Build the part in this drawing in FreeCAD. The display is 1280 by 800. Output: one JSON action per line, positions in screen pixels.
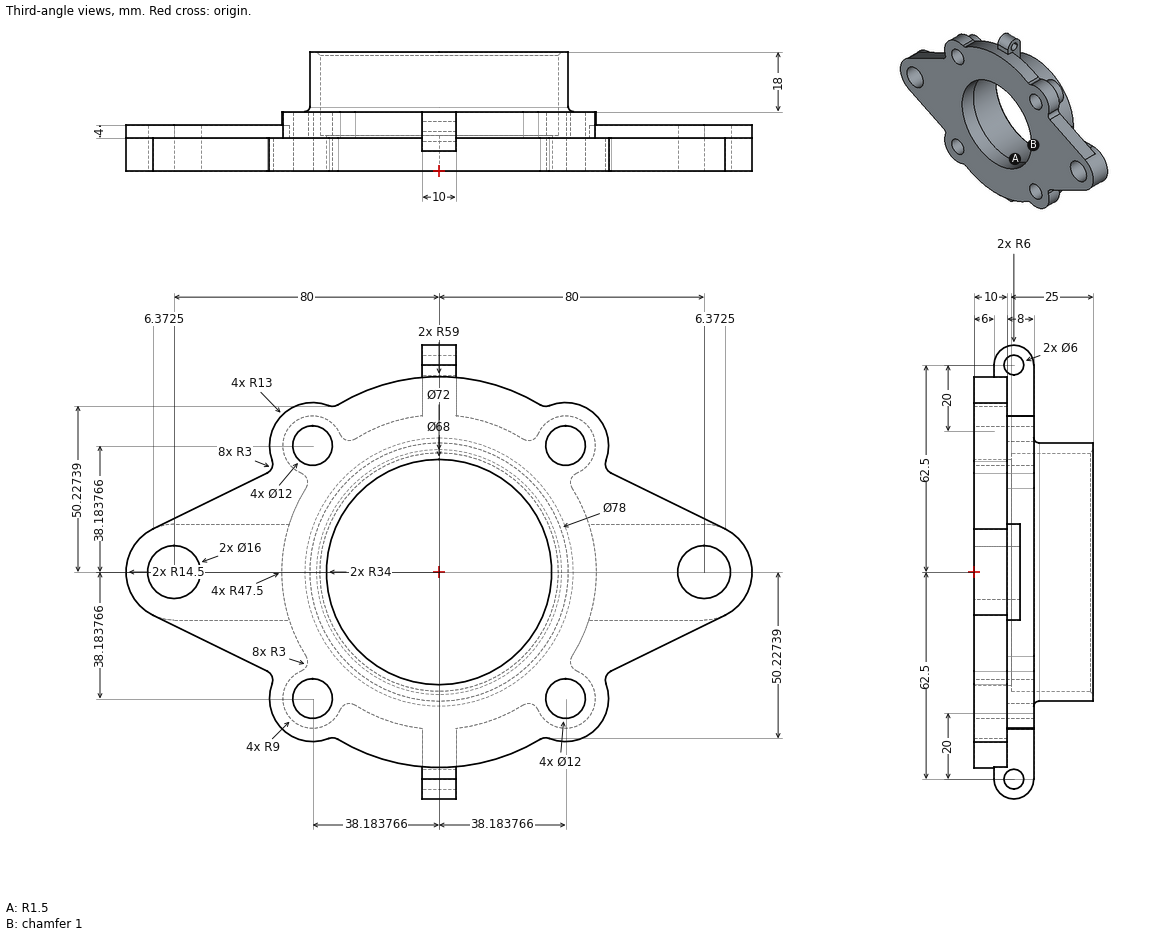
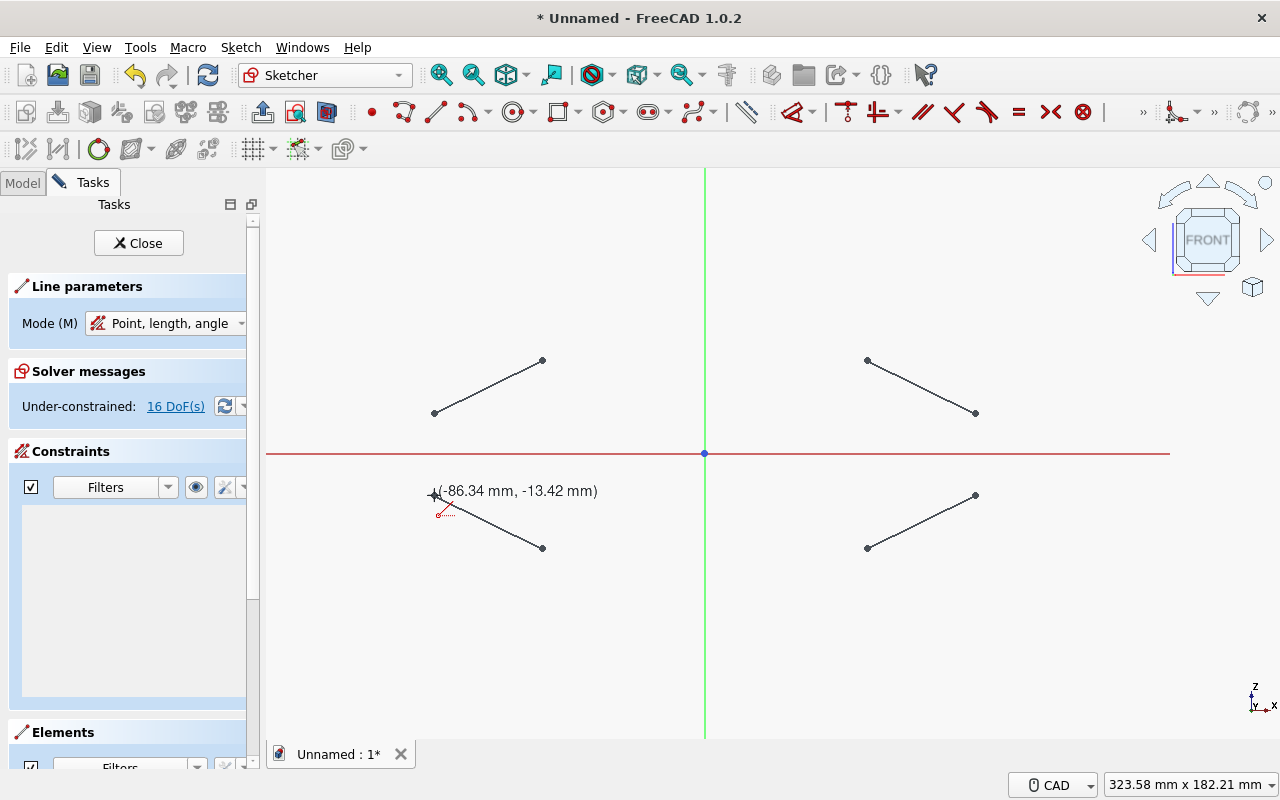
{"action": "left_click", "coordinate": [490, 112]}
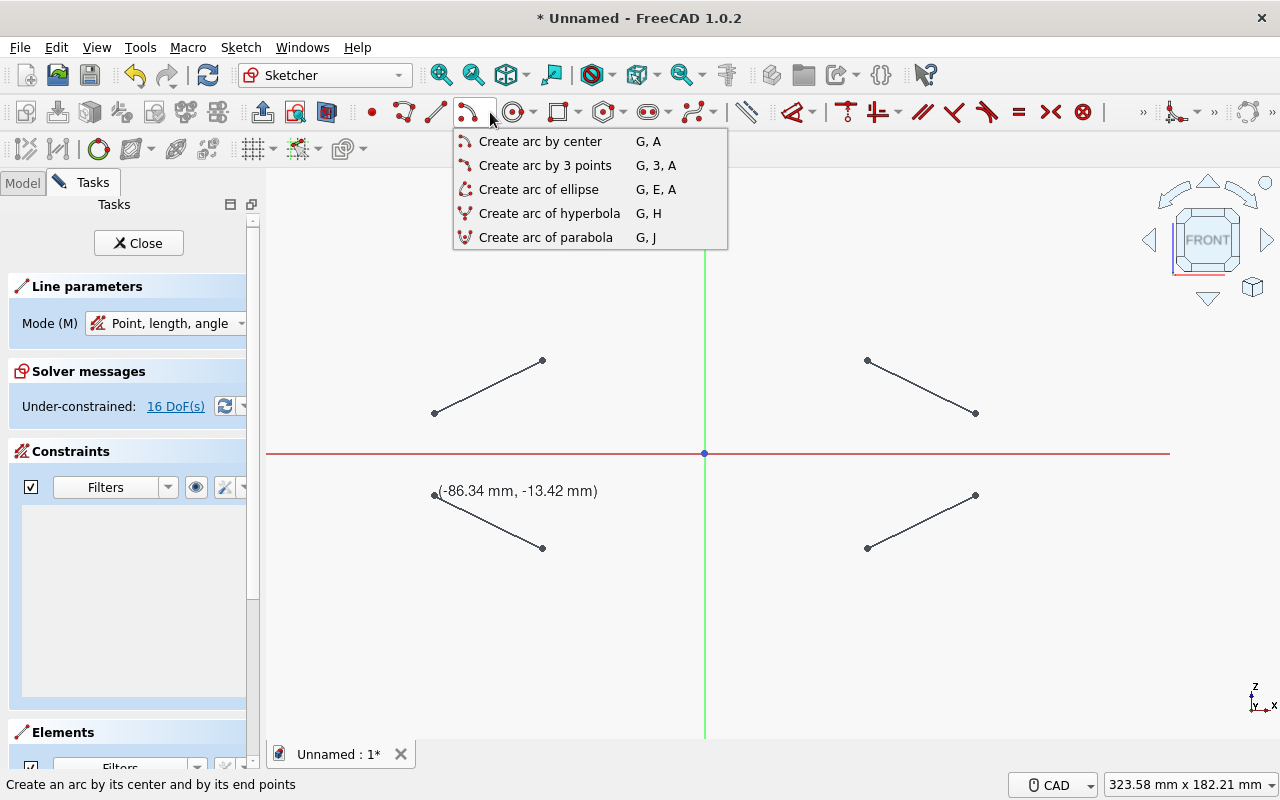
{"action": "left_click", "coordinate": [590, 165]}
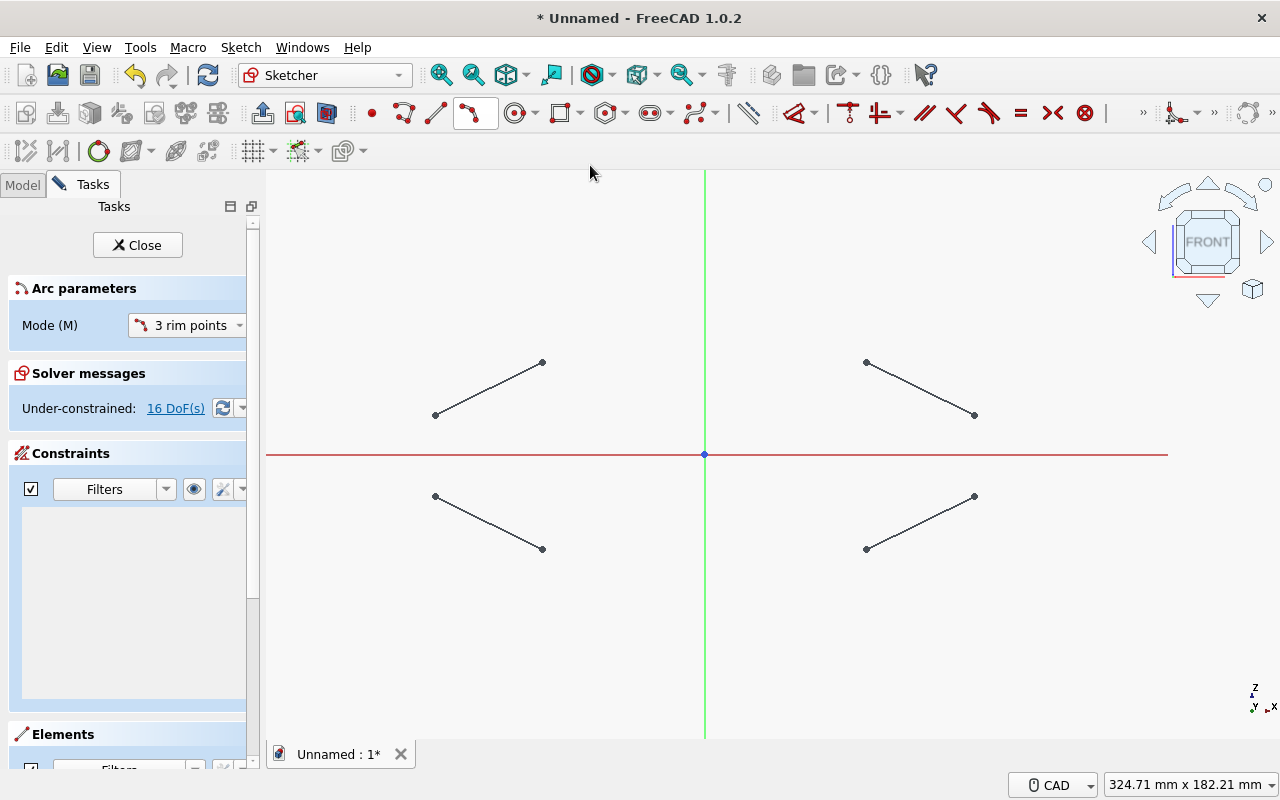
{"action": "left_click", "coordinate": [543, 362]}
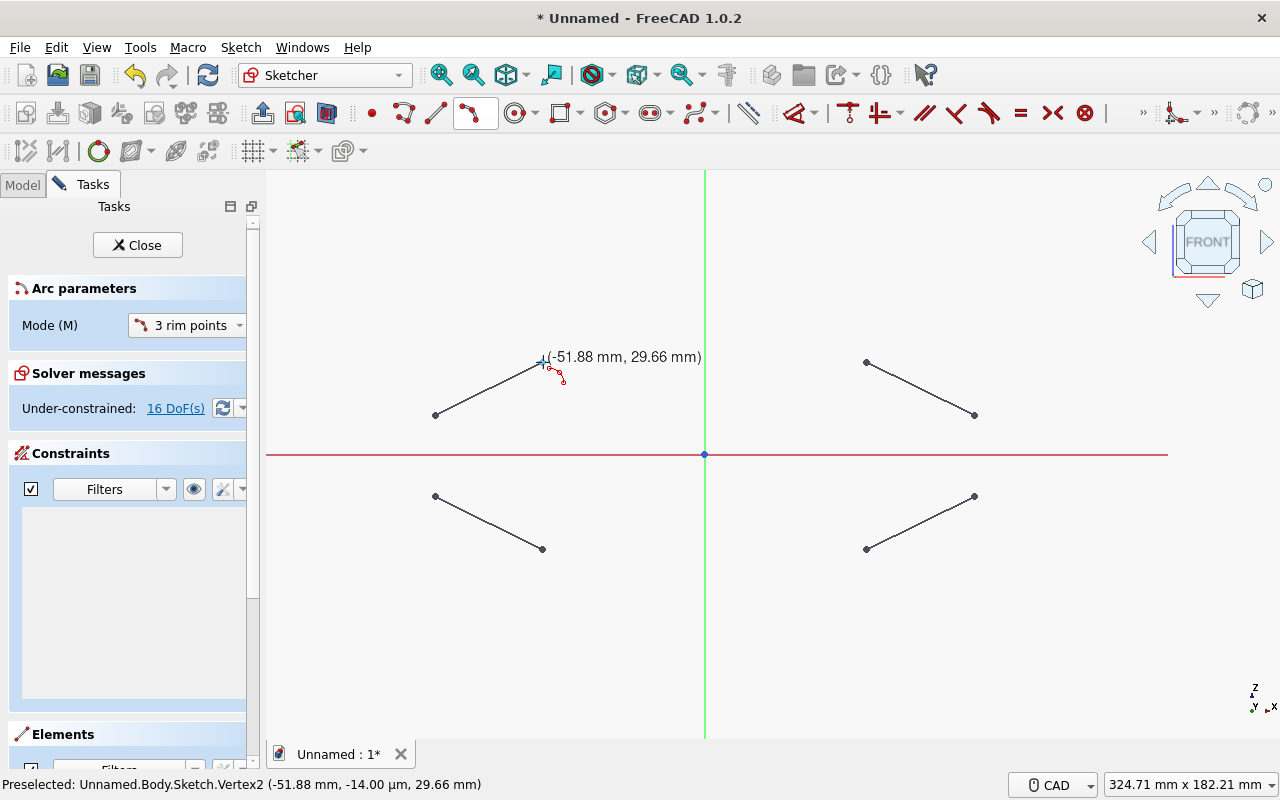
{"action": "scroll", "coordinate": [548, 350], "scroll_direction": "up", "scroll_amount": 2}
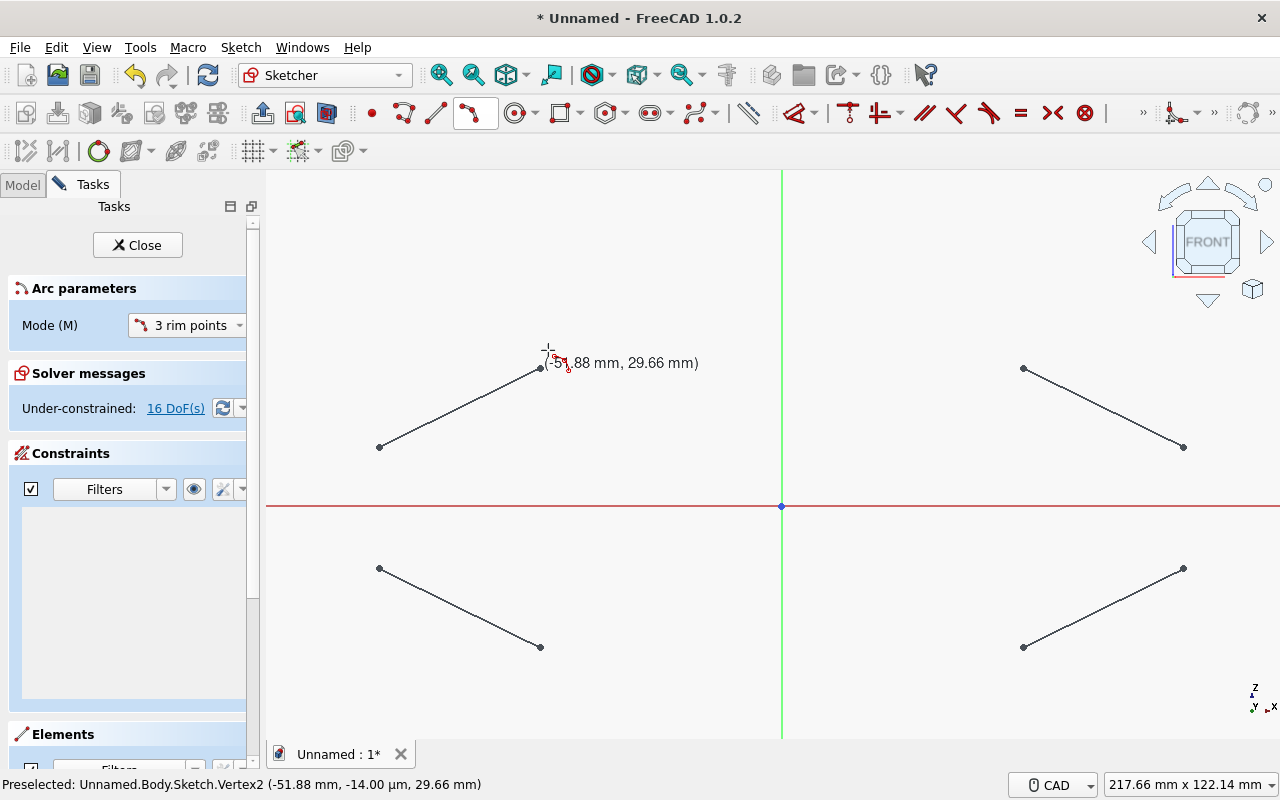
{"action": "left_click", "coordinate": [547, 350]}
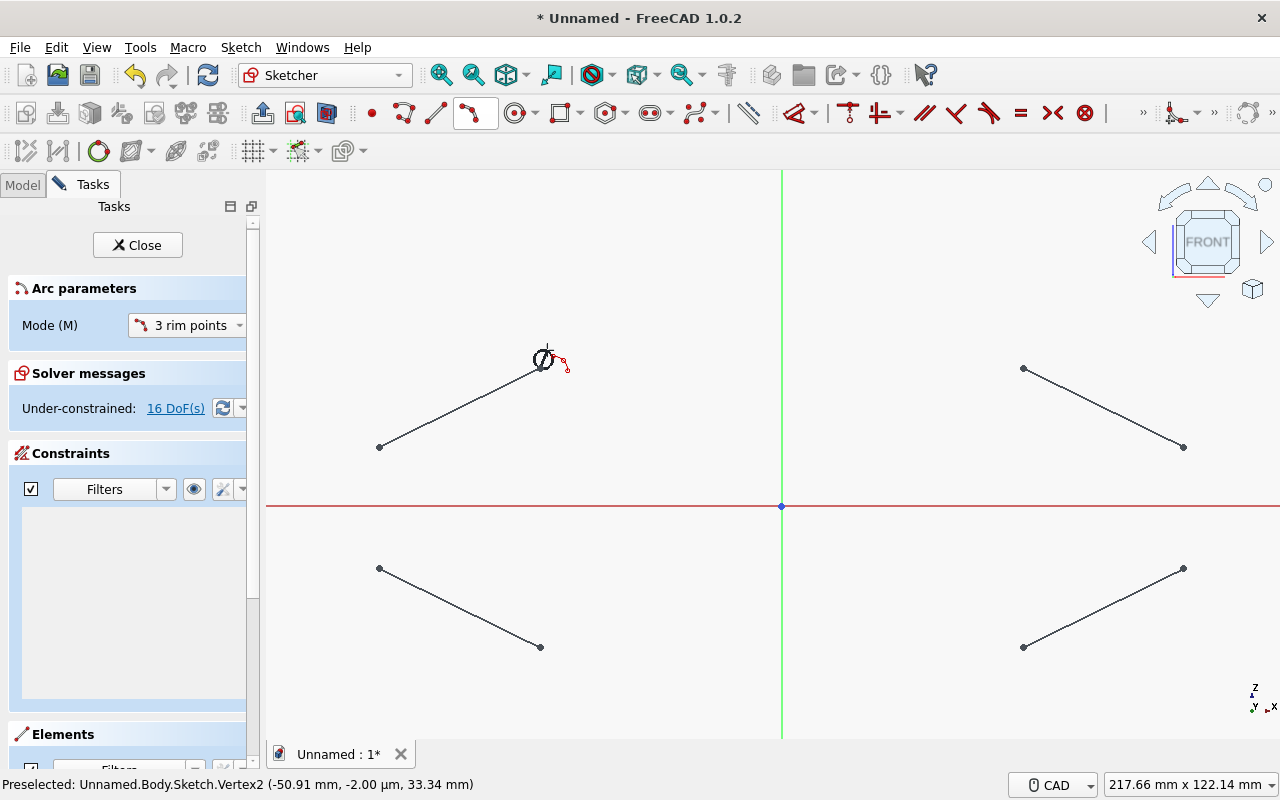
{"action": "scroll", "coordinate": [547, 360], "scroll_direction": "up", "scroll_amount": 8}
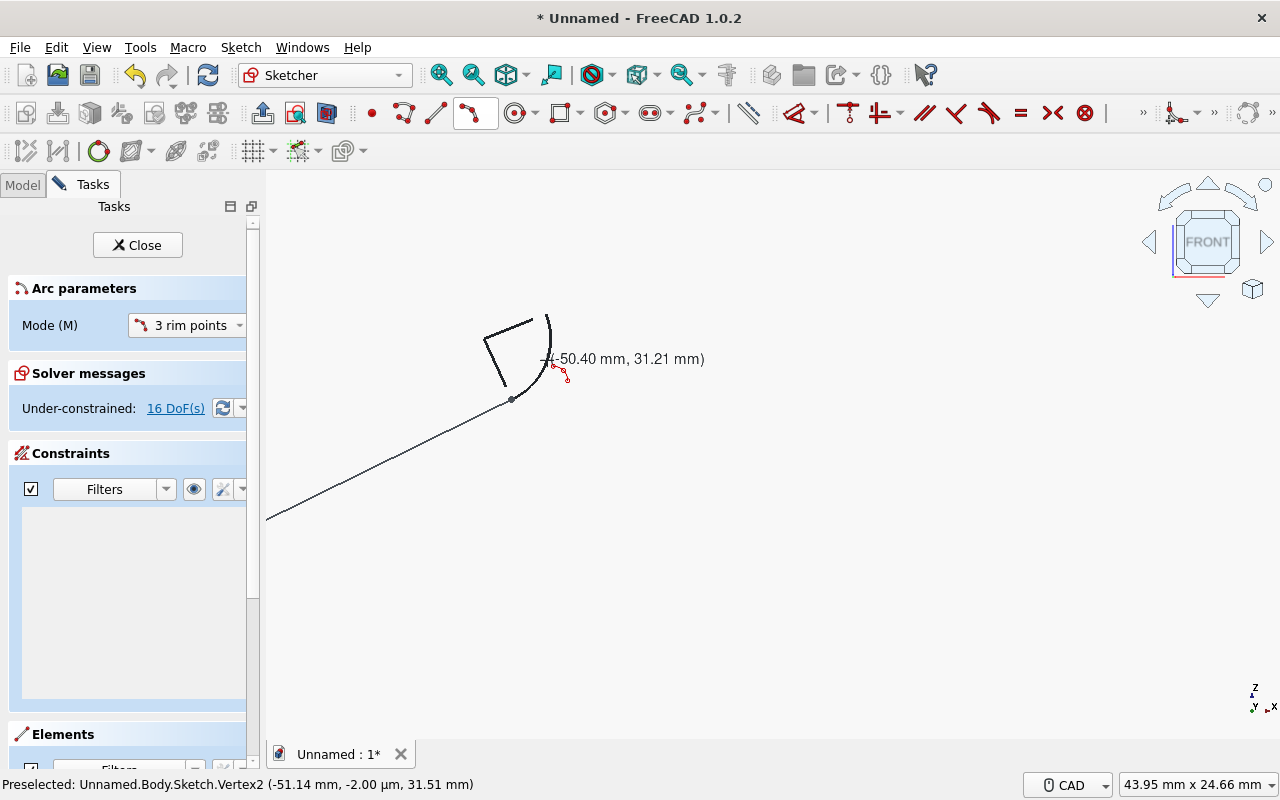
{"action": "left_click", "coordinate": [546, 357]}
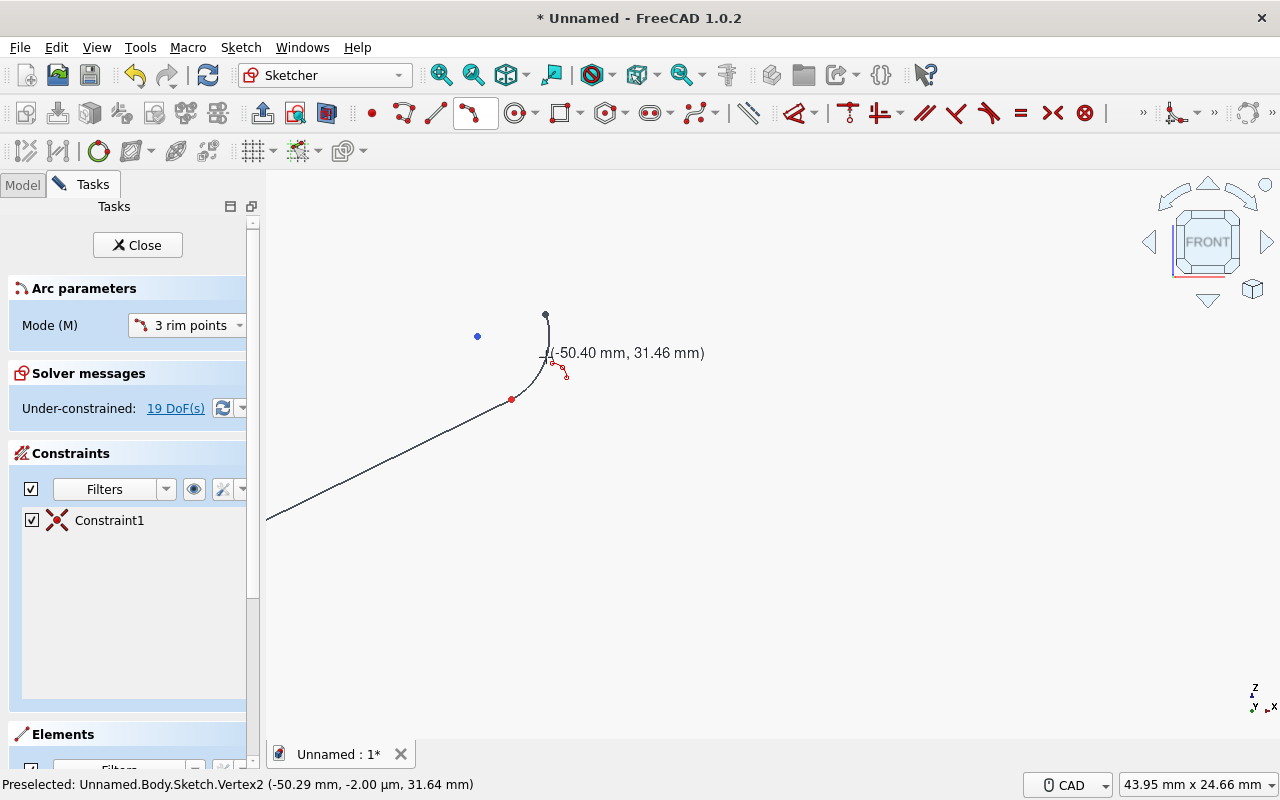
{"action": "scroll", "coordinate": [547, 356], "scroll_direction": "down", "scroll_amount": 10}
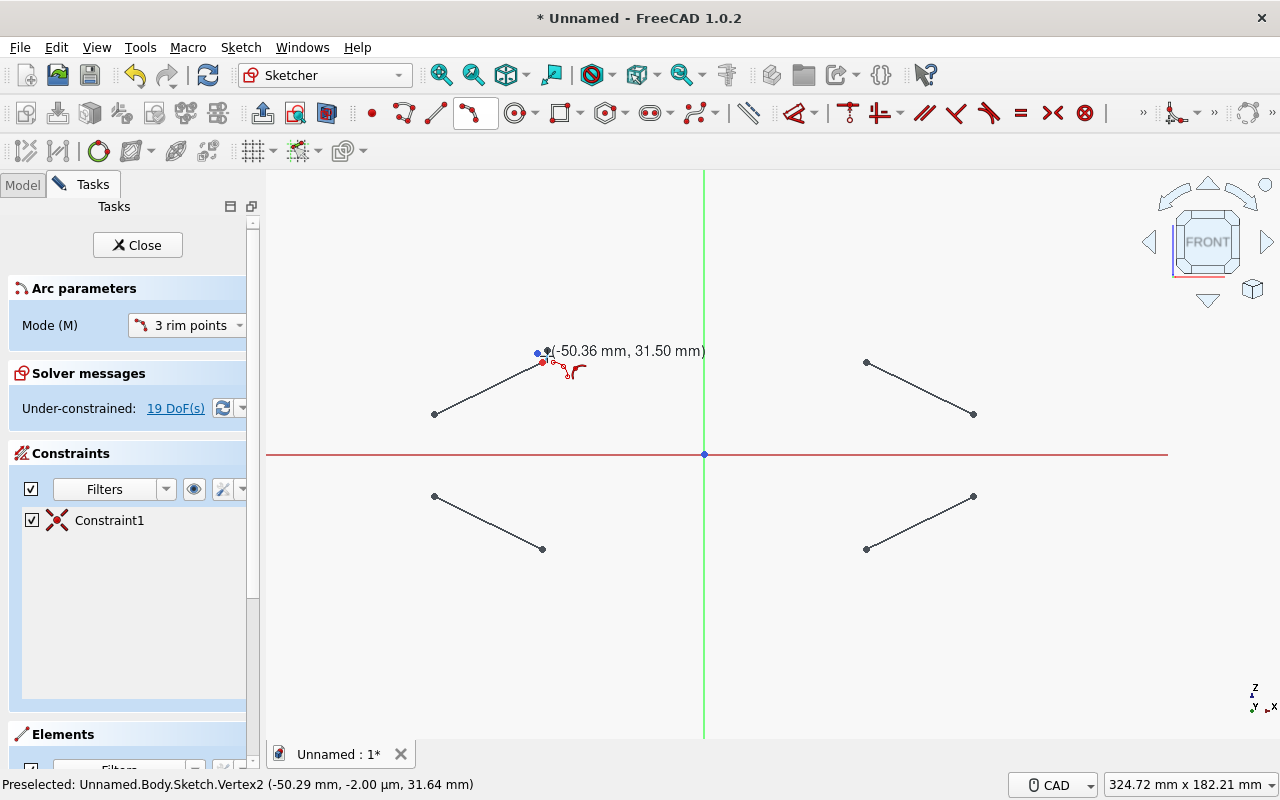
{"action": "scroll", "coordinate": [547, 350], "scroll_direction": "up", "scroll_amount": 3}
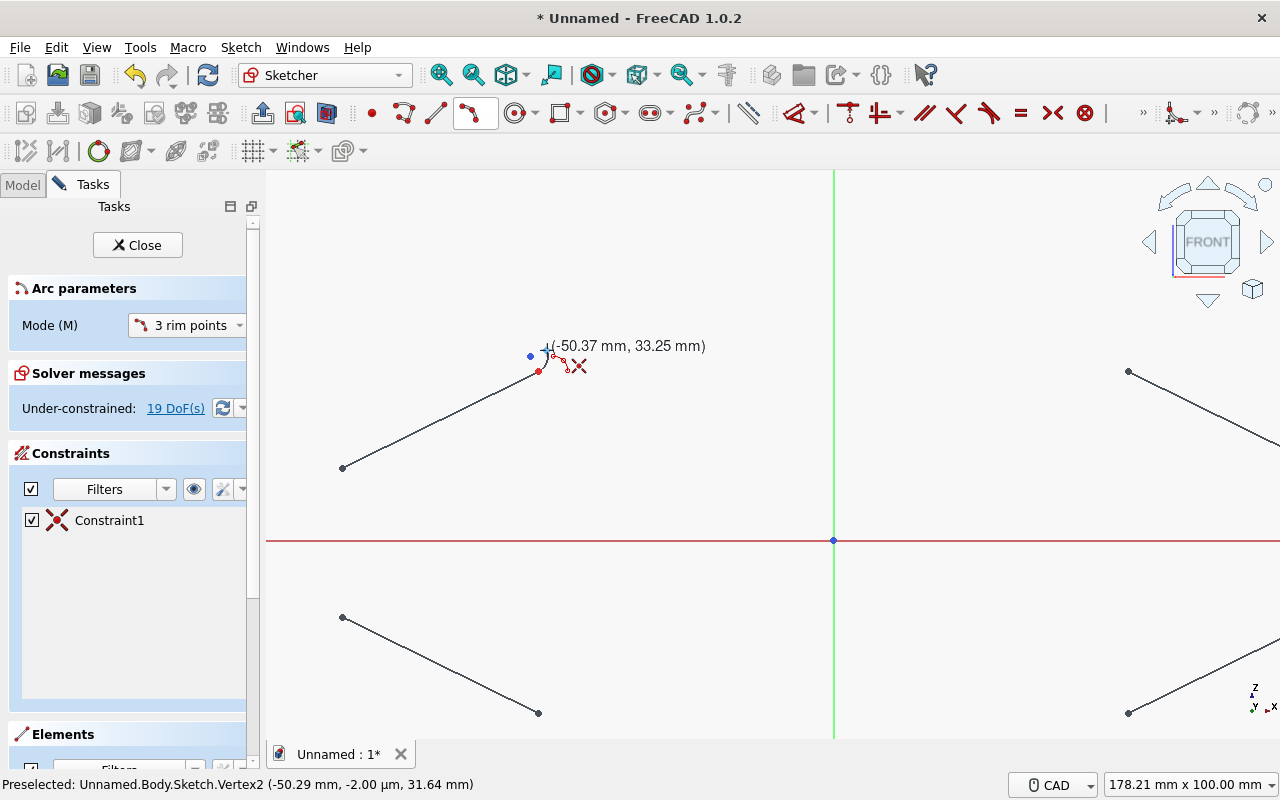
{"action": "left_click", "coordinate": [547, 351]}
{"action": "left_click", "coordinate": [644, 255]}
{"action": "left_click", "coordinate": [565, 270]}